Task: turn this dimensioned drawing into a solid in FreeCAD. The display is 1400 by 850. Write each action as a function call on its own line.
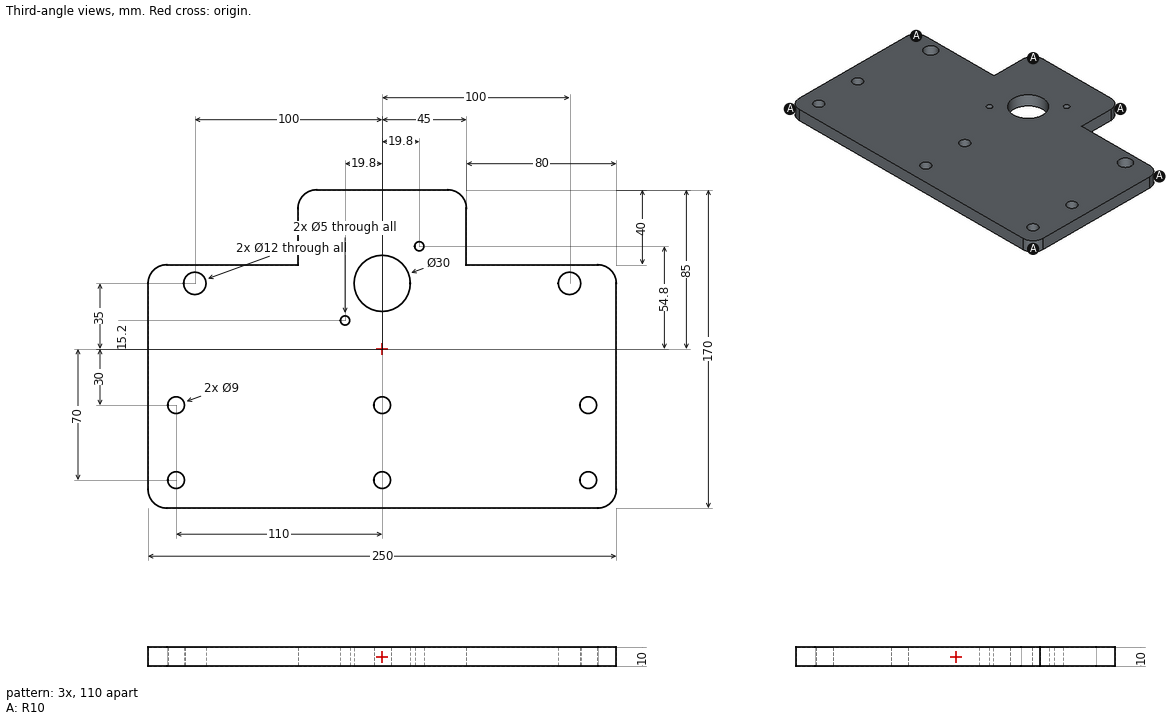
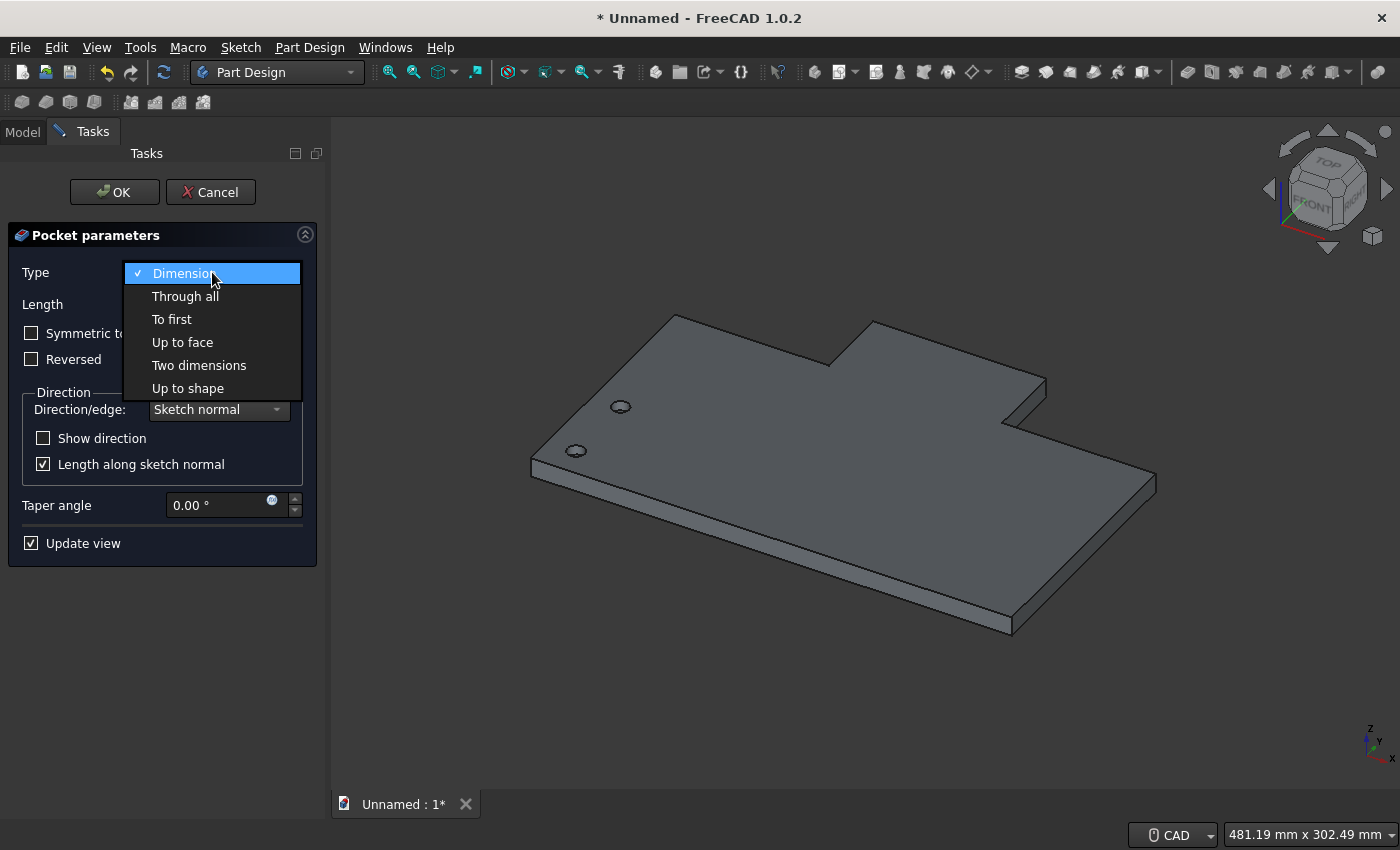
click(212, 296)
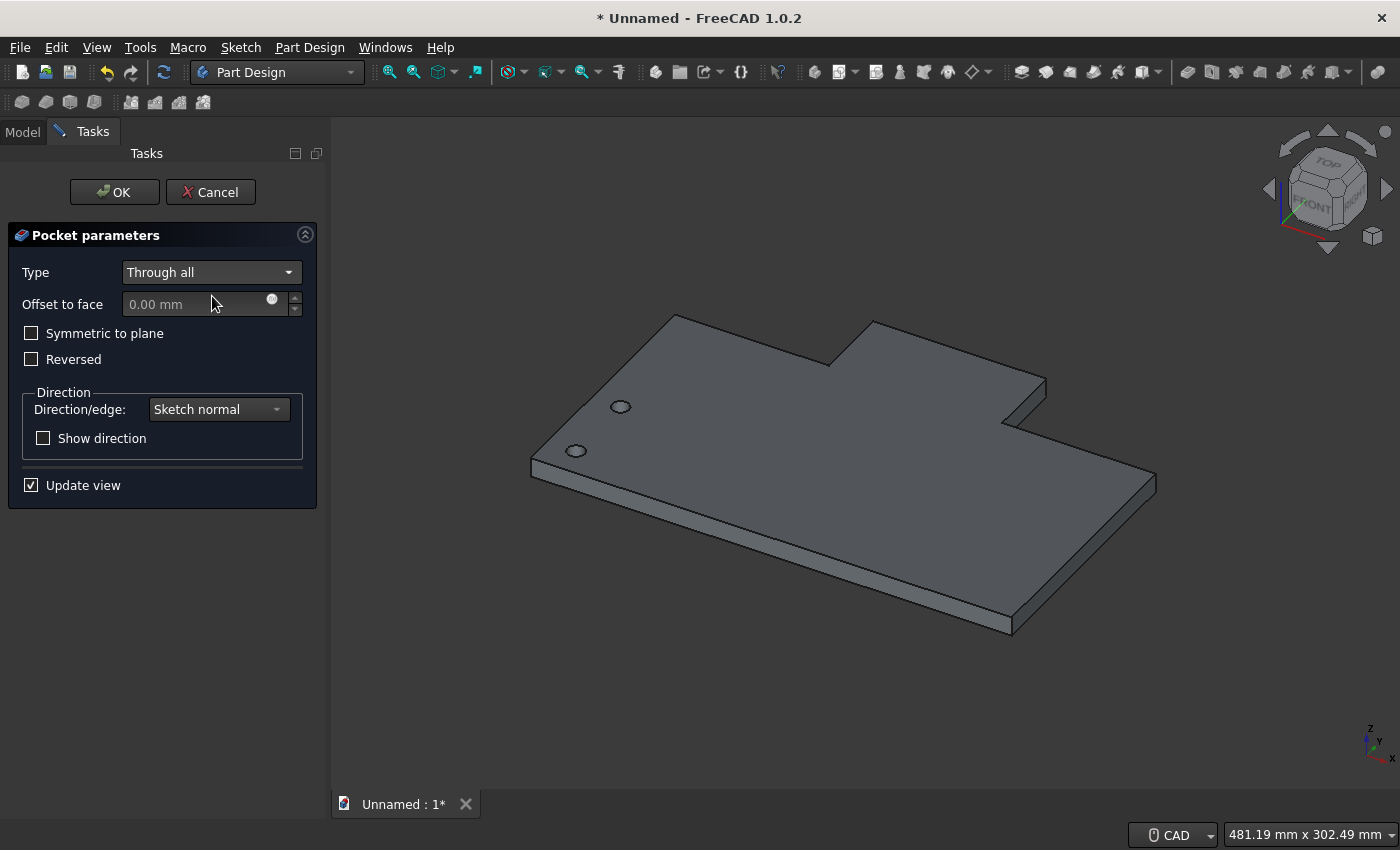
click(115, 192)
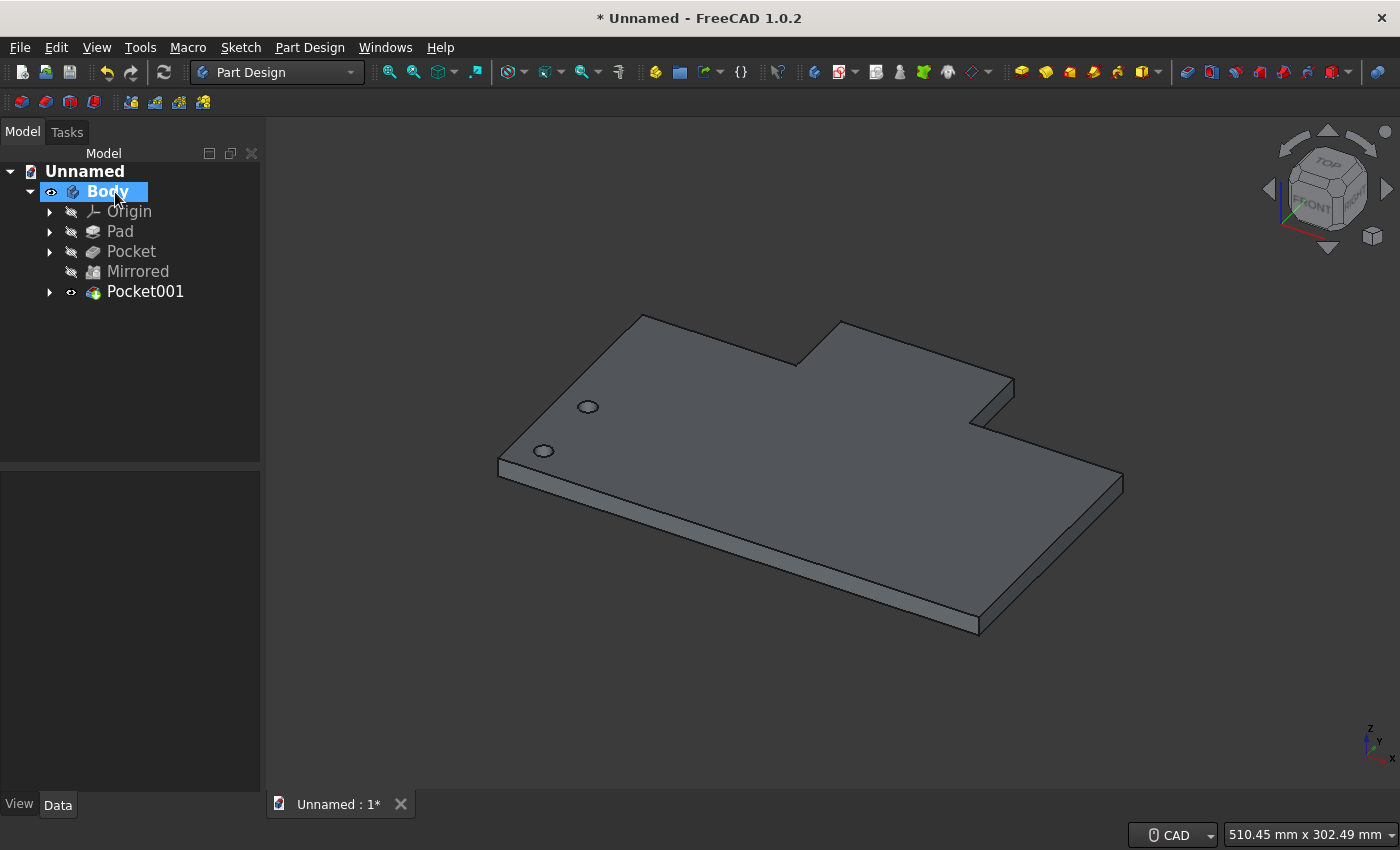
click(116, 292)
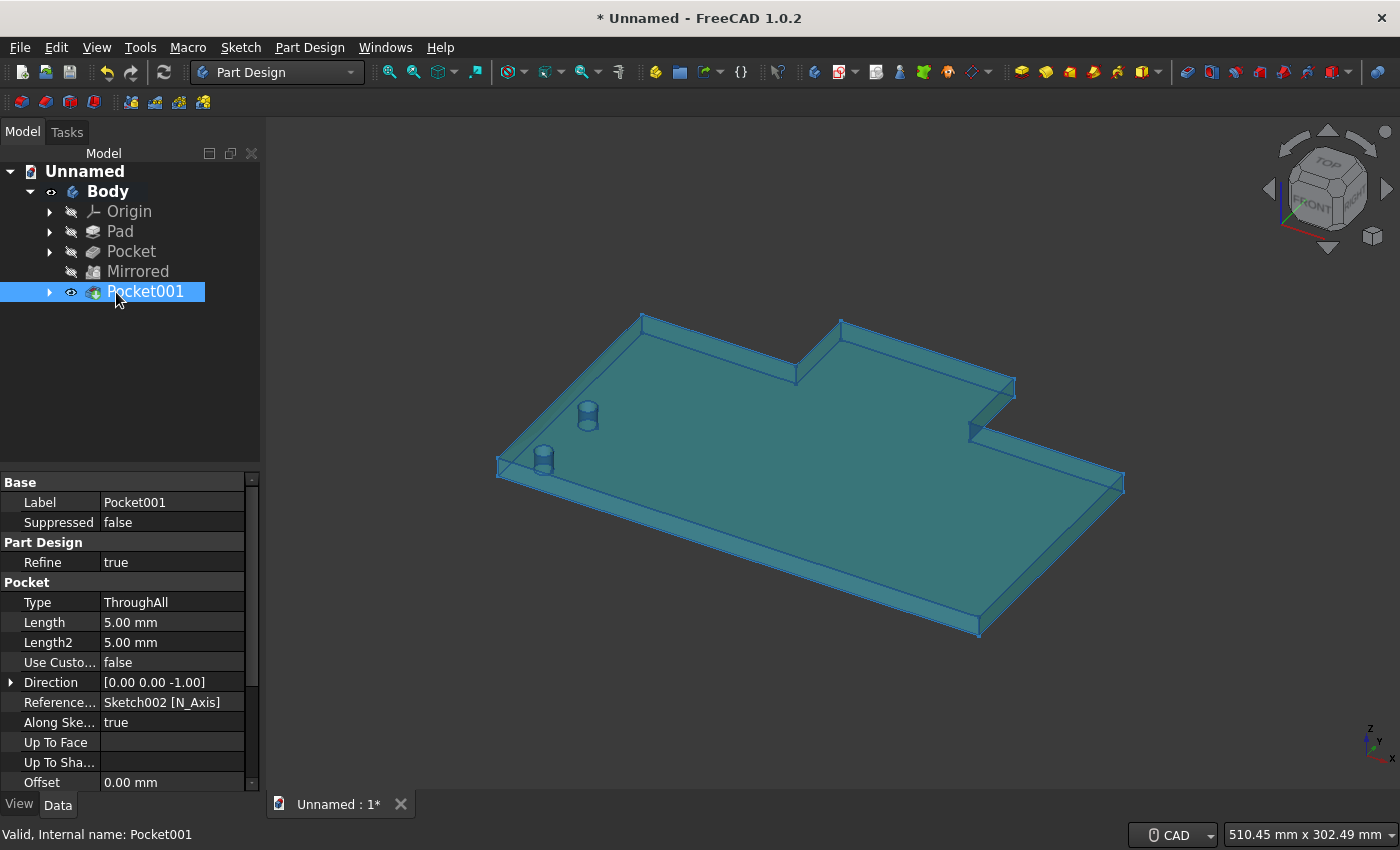
click(156, 102)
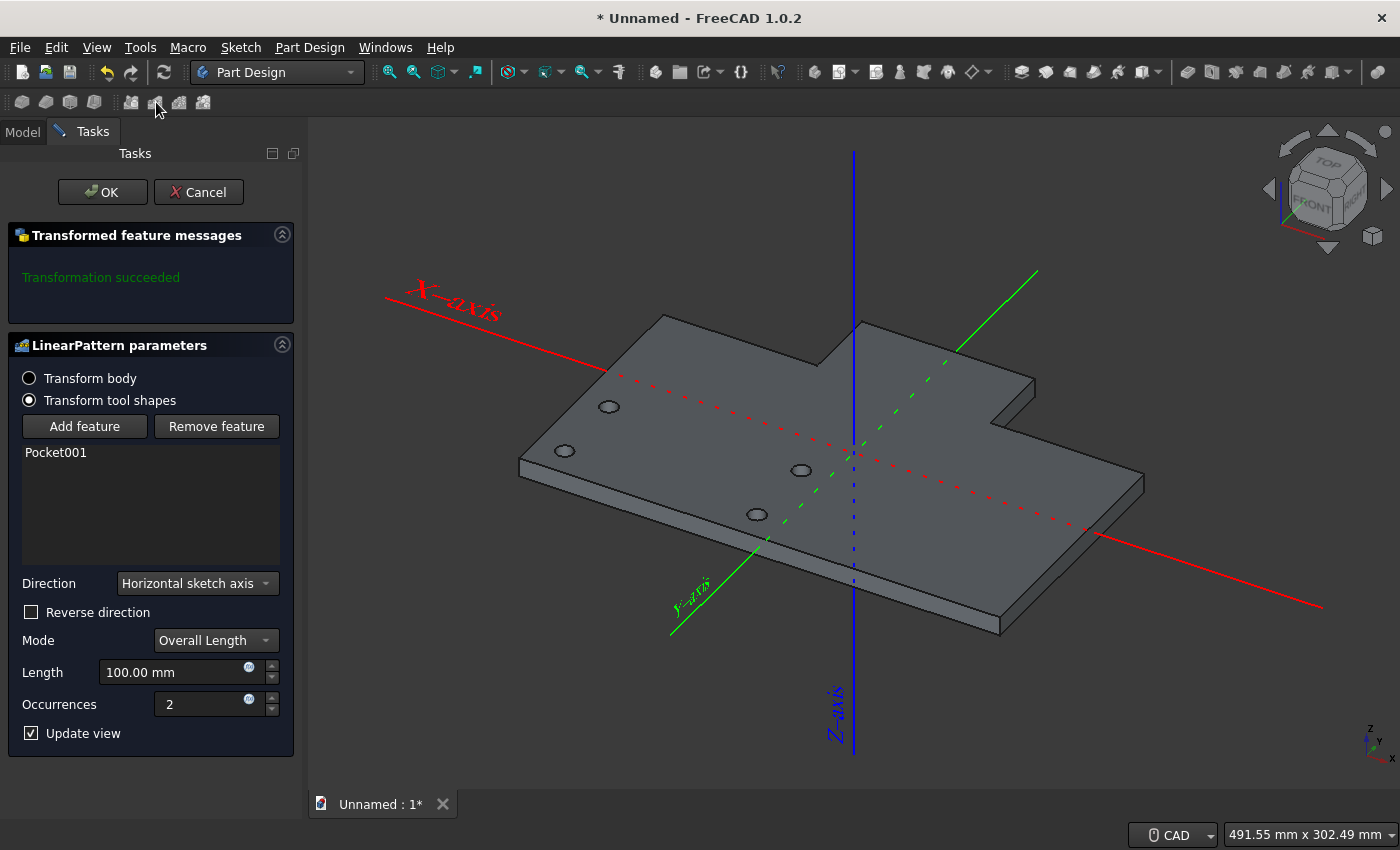
click(198, 584)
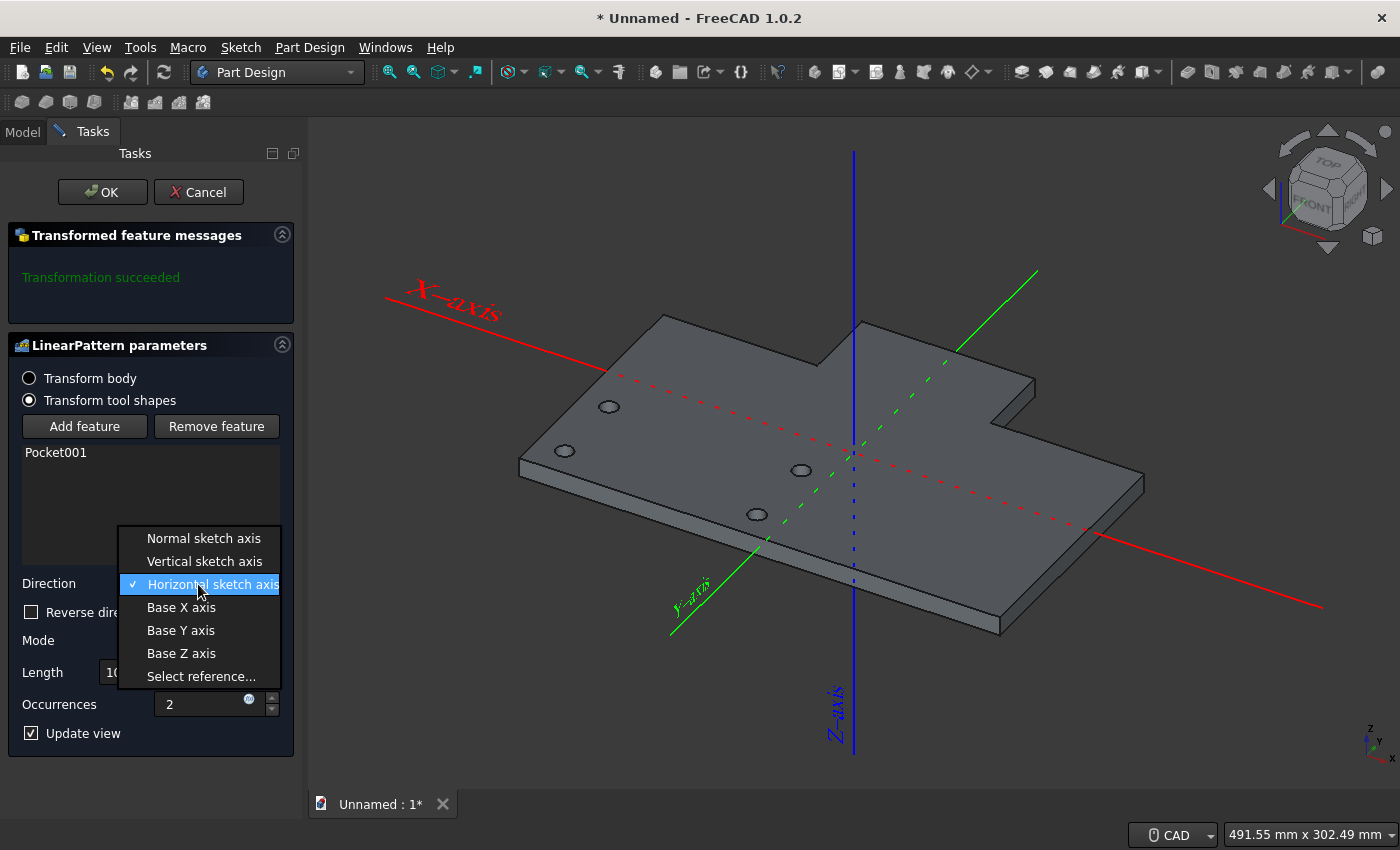
click(198, 608)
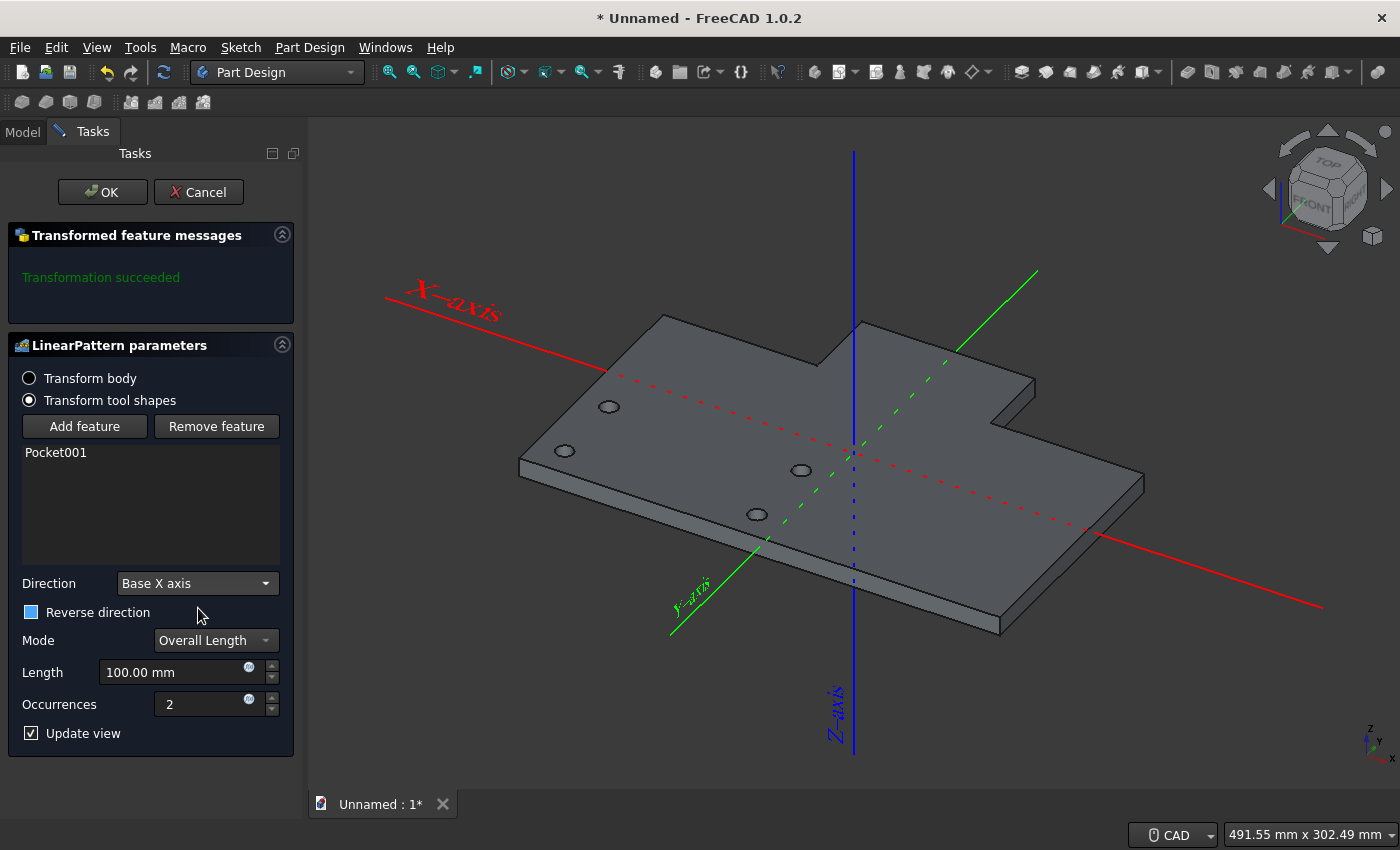
click(217, 640)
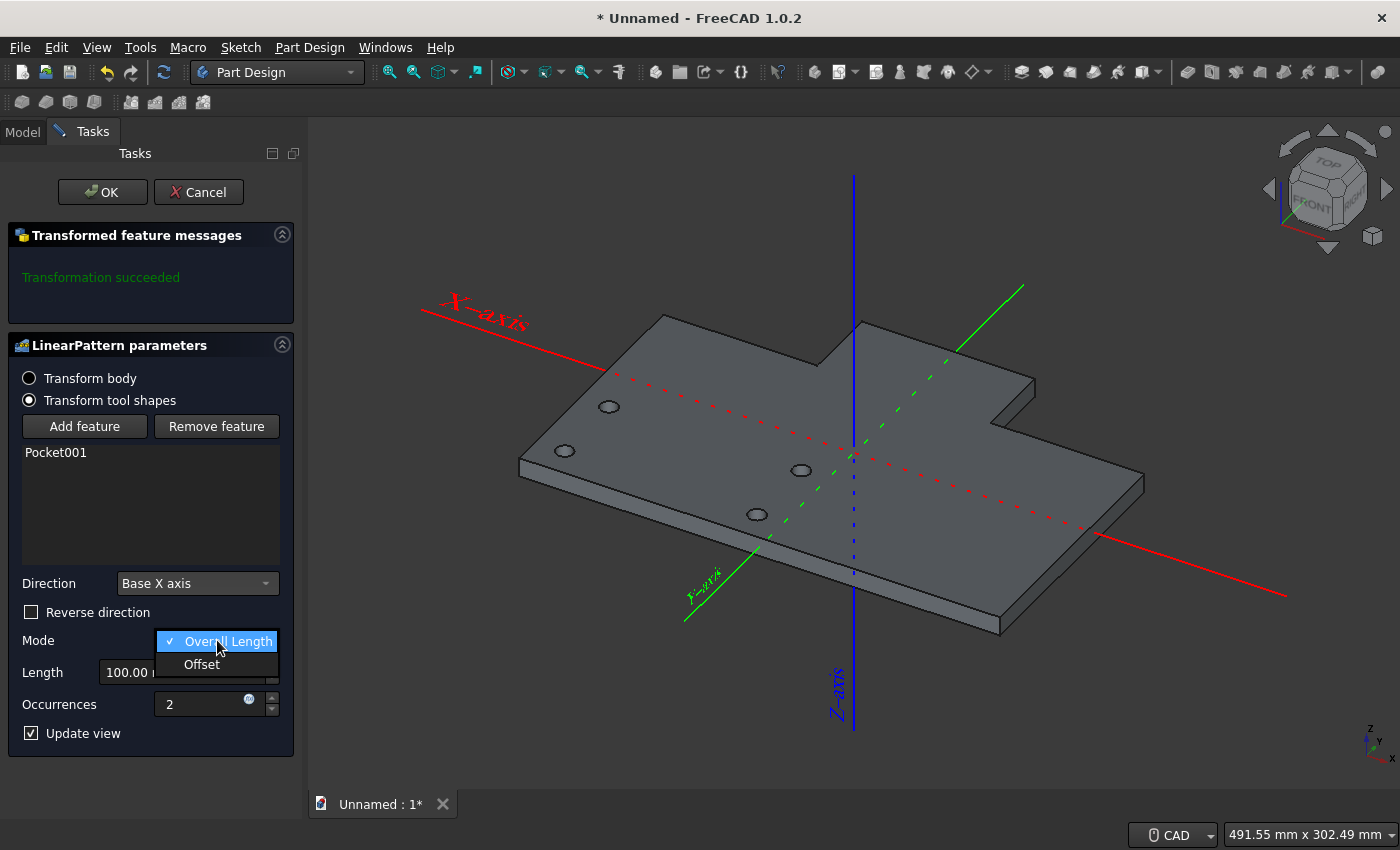
click(216, 664)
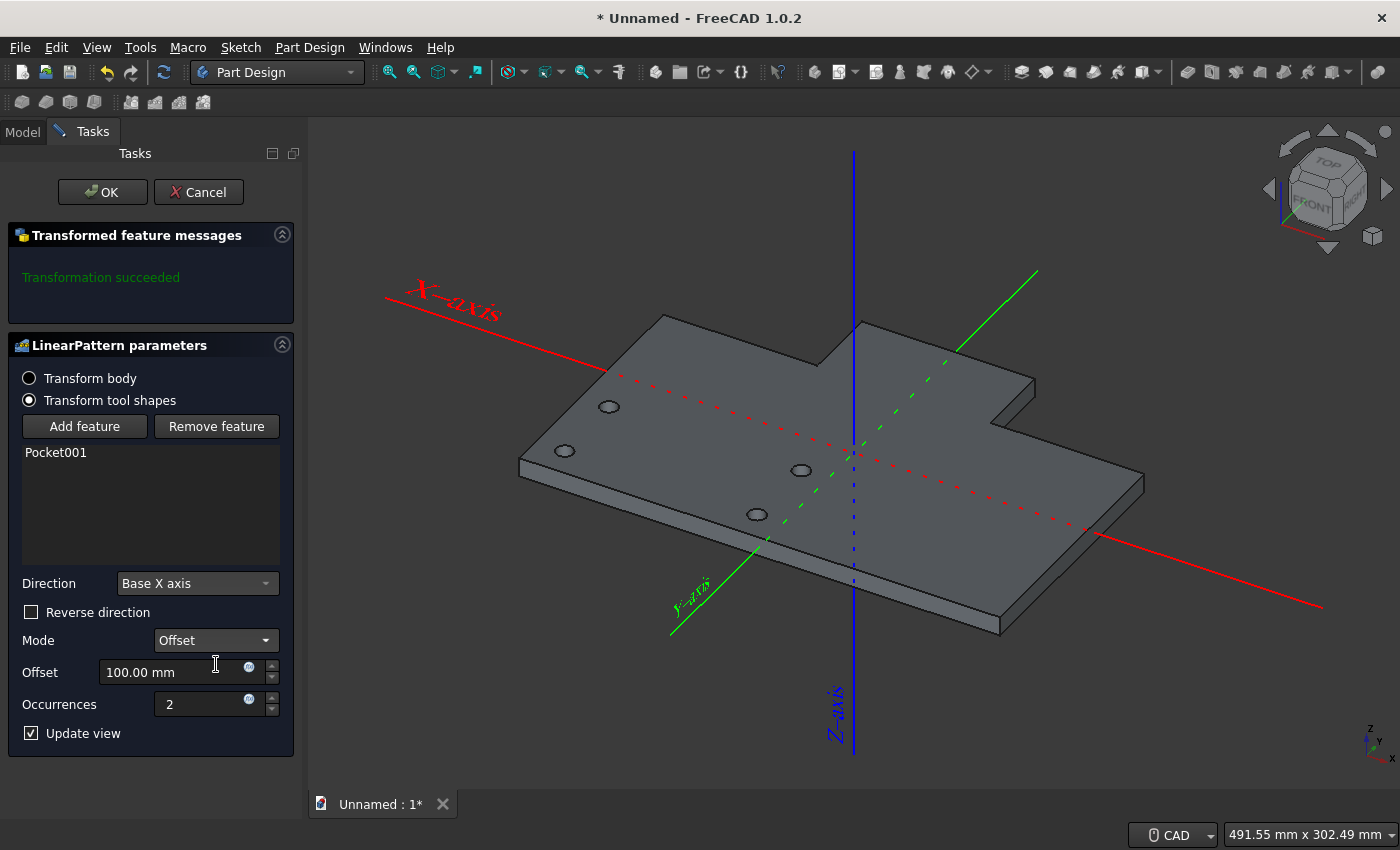
triple_click(182, 672)